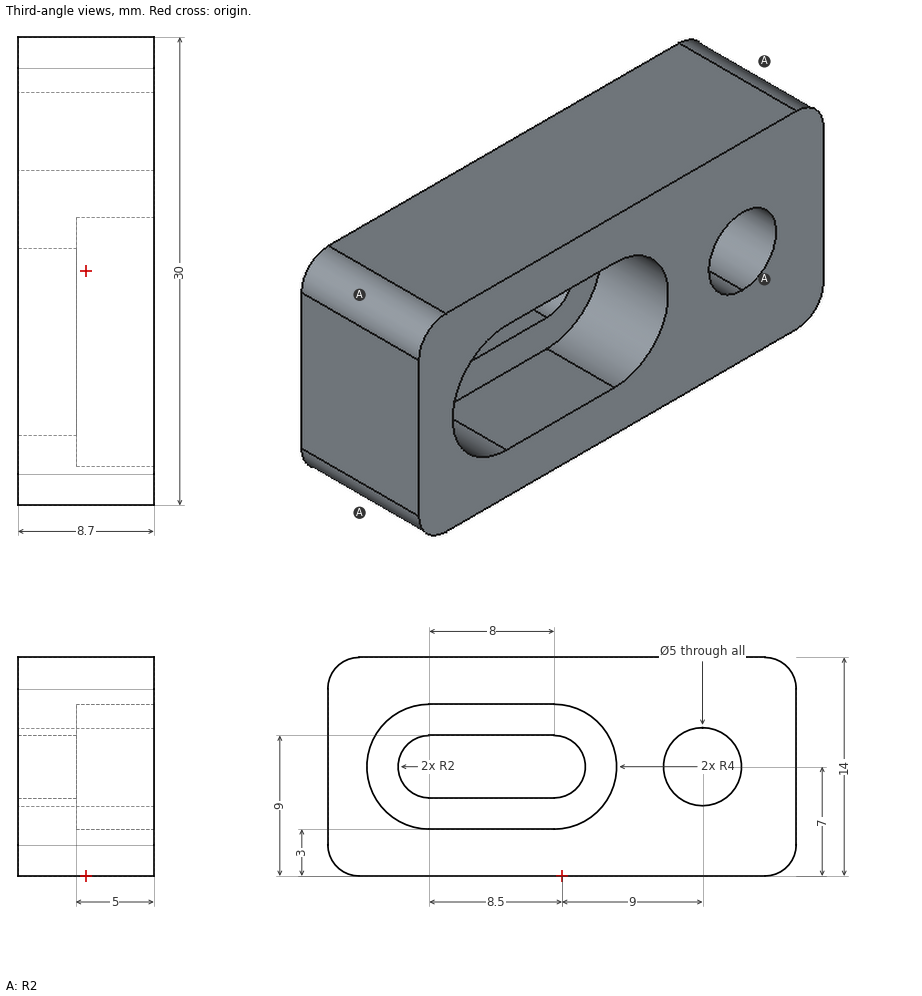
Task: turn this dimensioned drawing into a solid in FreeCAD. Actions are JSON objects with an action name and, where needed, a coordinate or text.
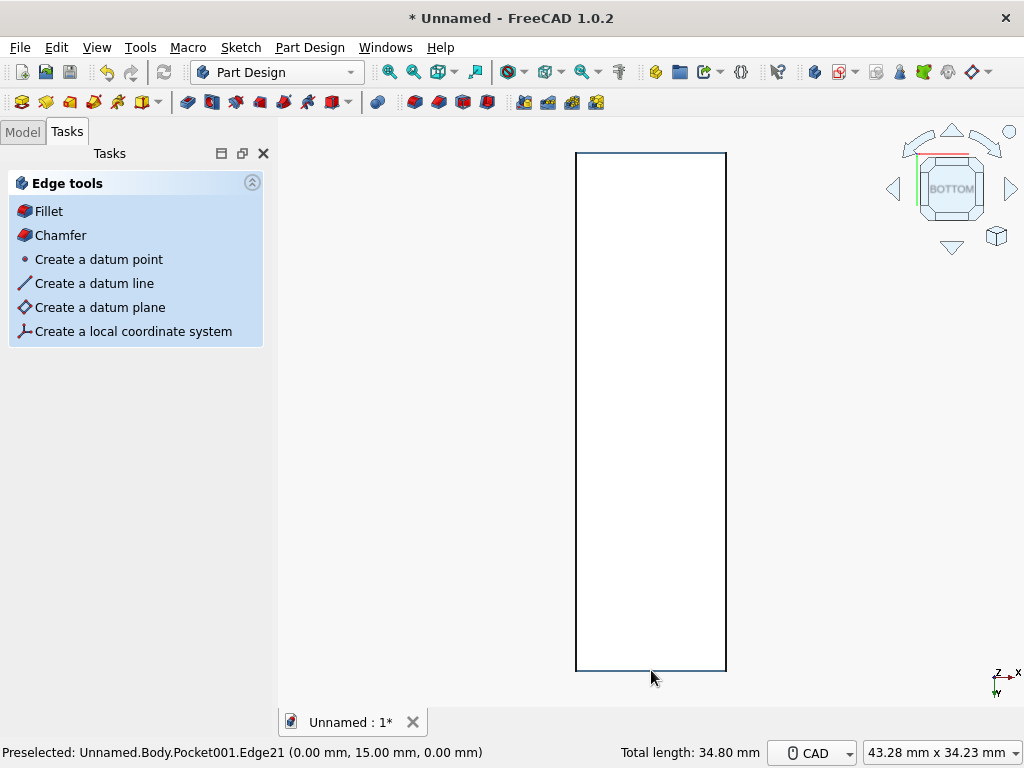
{"action": "left_click", "coordinate": [416, 102]}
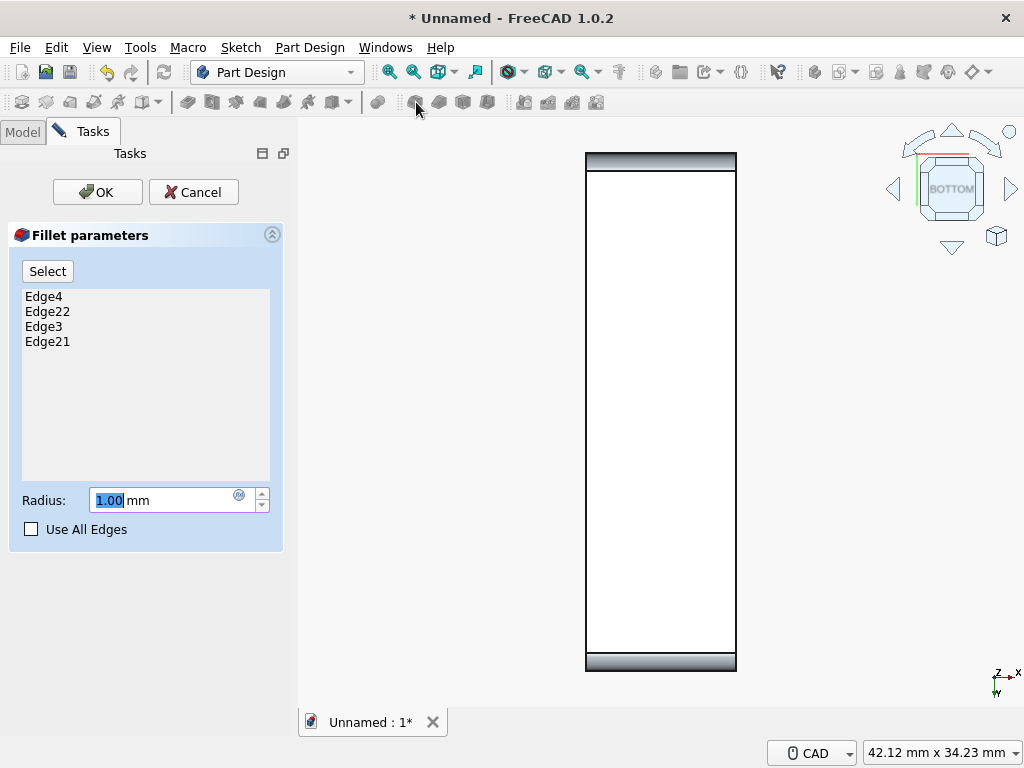
{"action": "type", "text": "2"}
{"action": "key", "text": "Tab"}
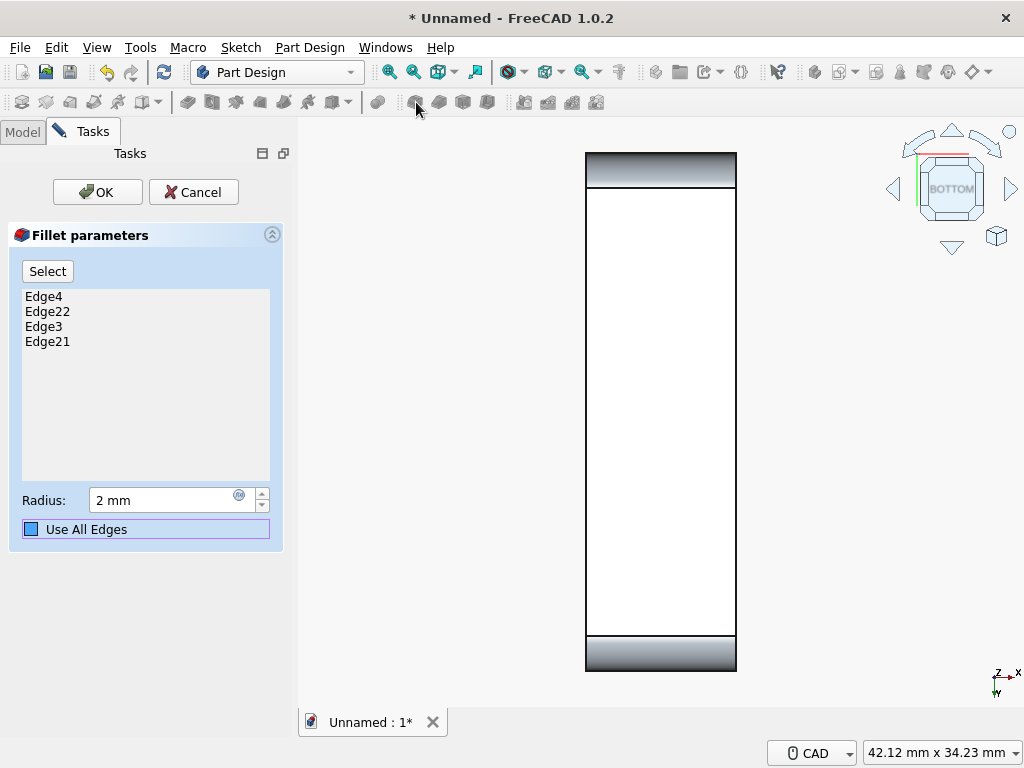
{"action": "left_click", "coordinate": [98, 192]}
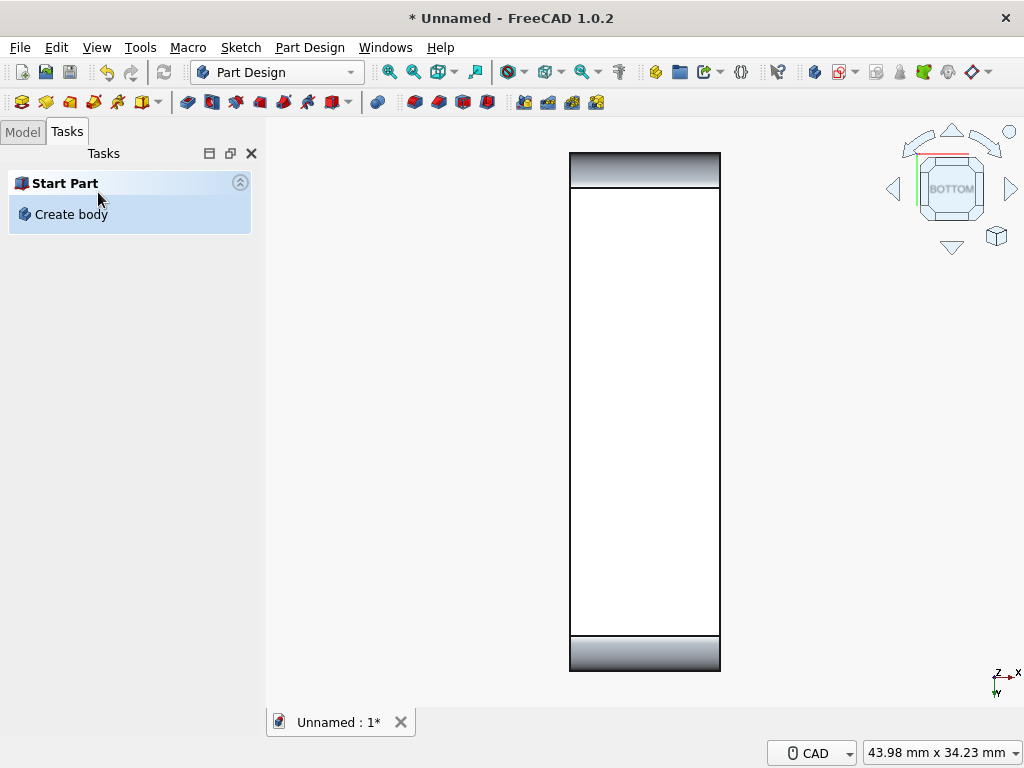
{"action": "key", "text": "0"}